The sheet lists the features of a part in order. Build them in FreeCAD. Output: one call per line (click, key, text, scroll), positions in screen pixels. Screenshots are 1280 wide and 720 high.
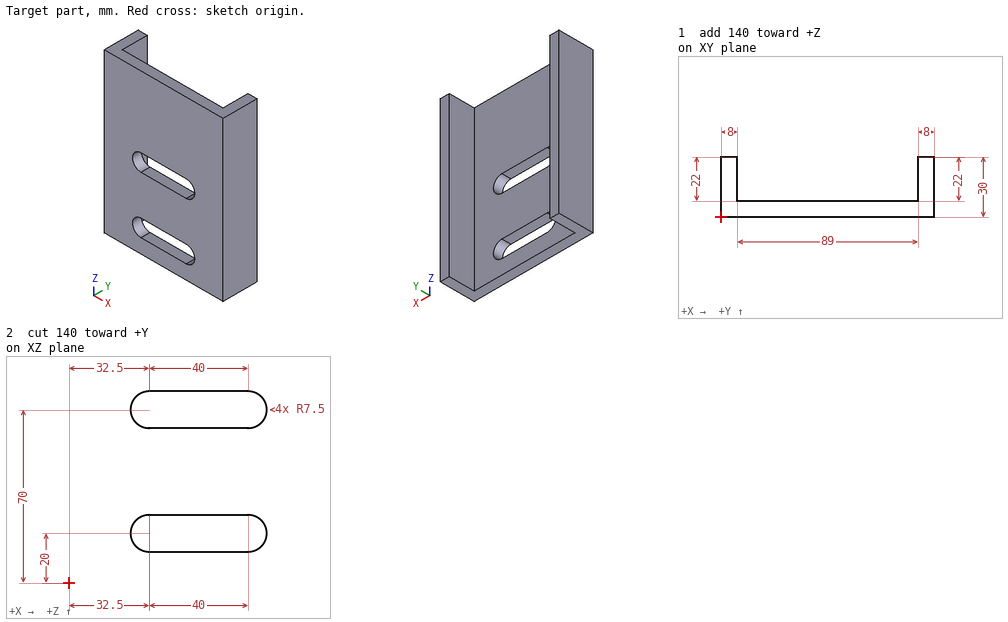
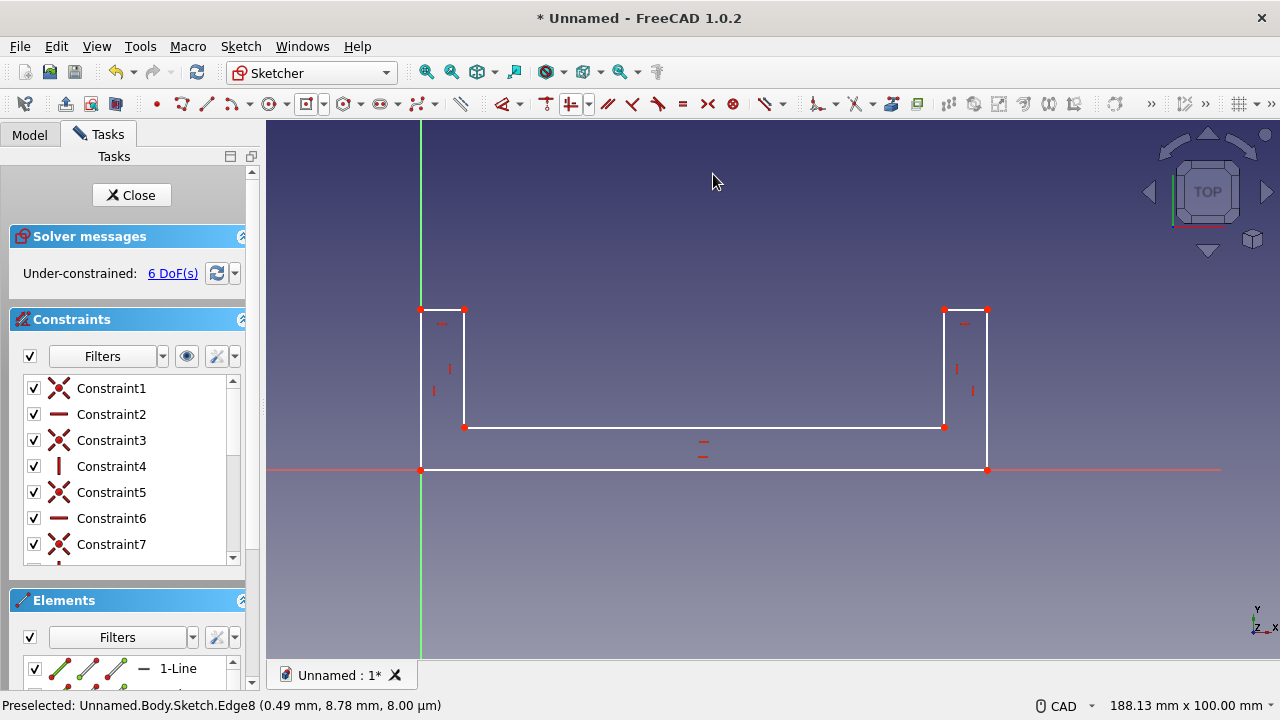
click(502, 104)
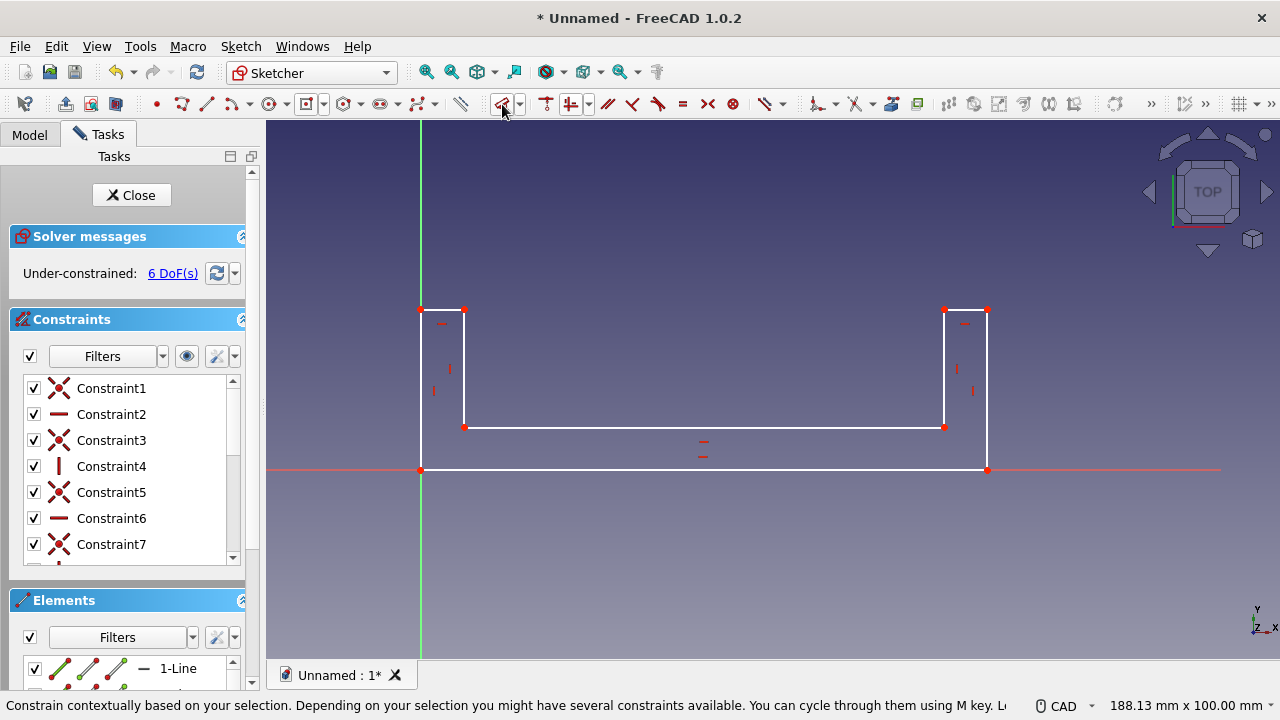
click(974, 310)
click(966, 276)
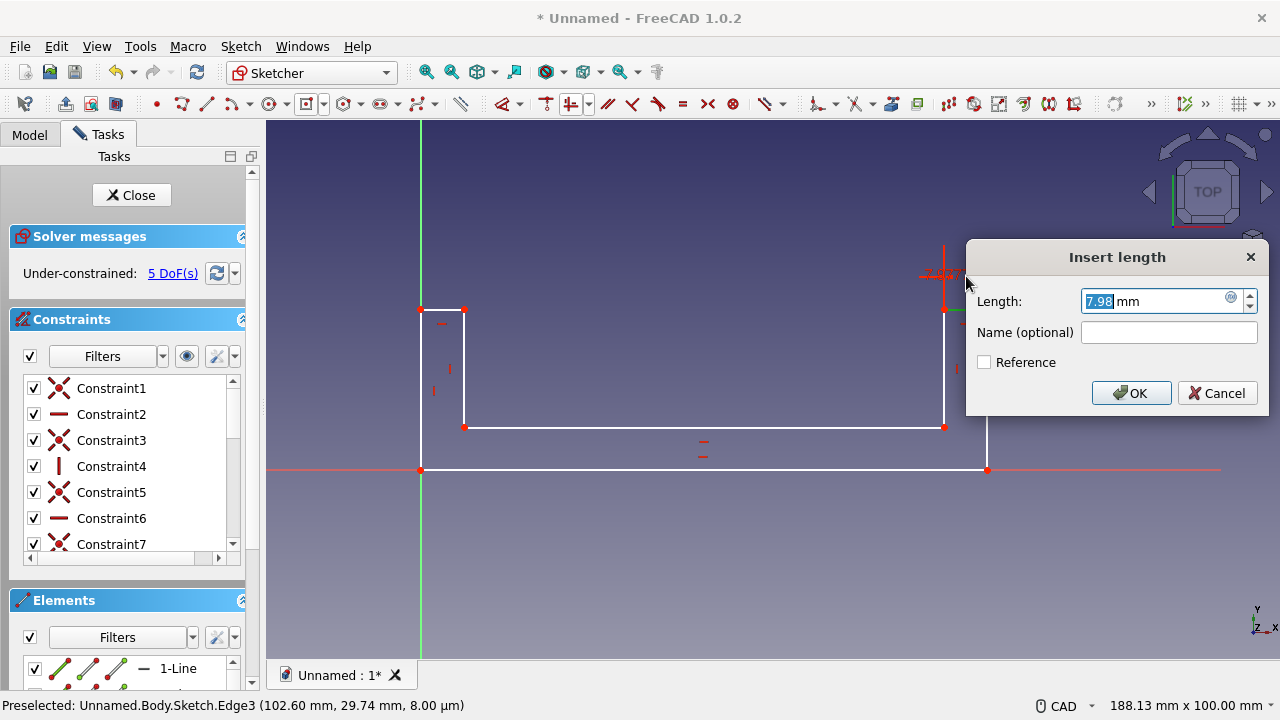
text(8)
key(Return)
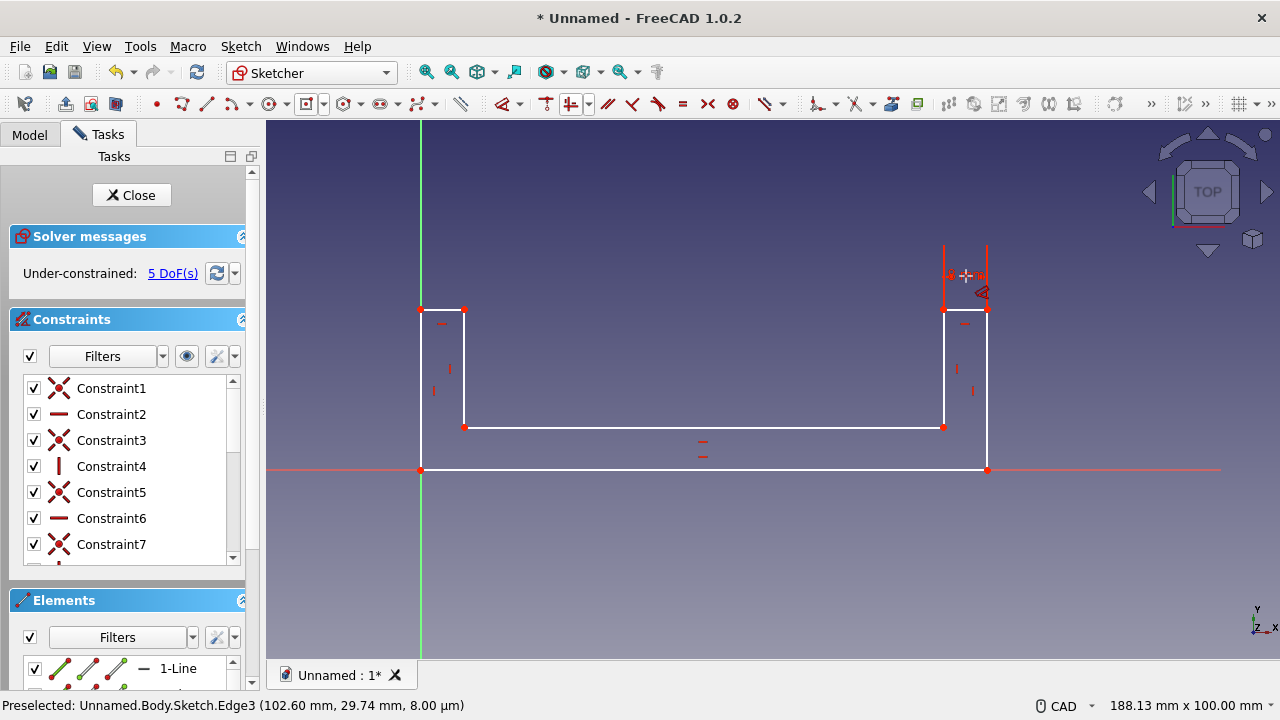
click(451, 310)
click(442, 276)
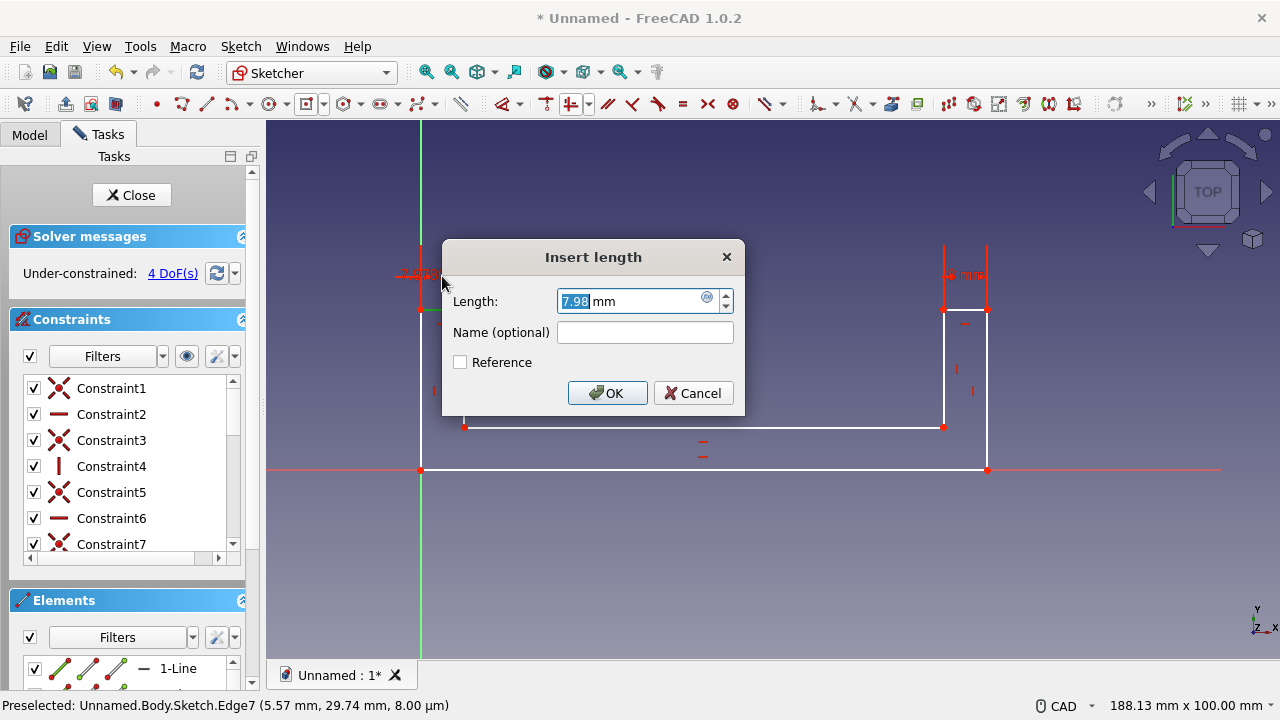
text(8)
key(Return)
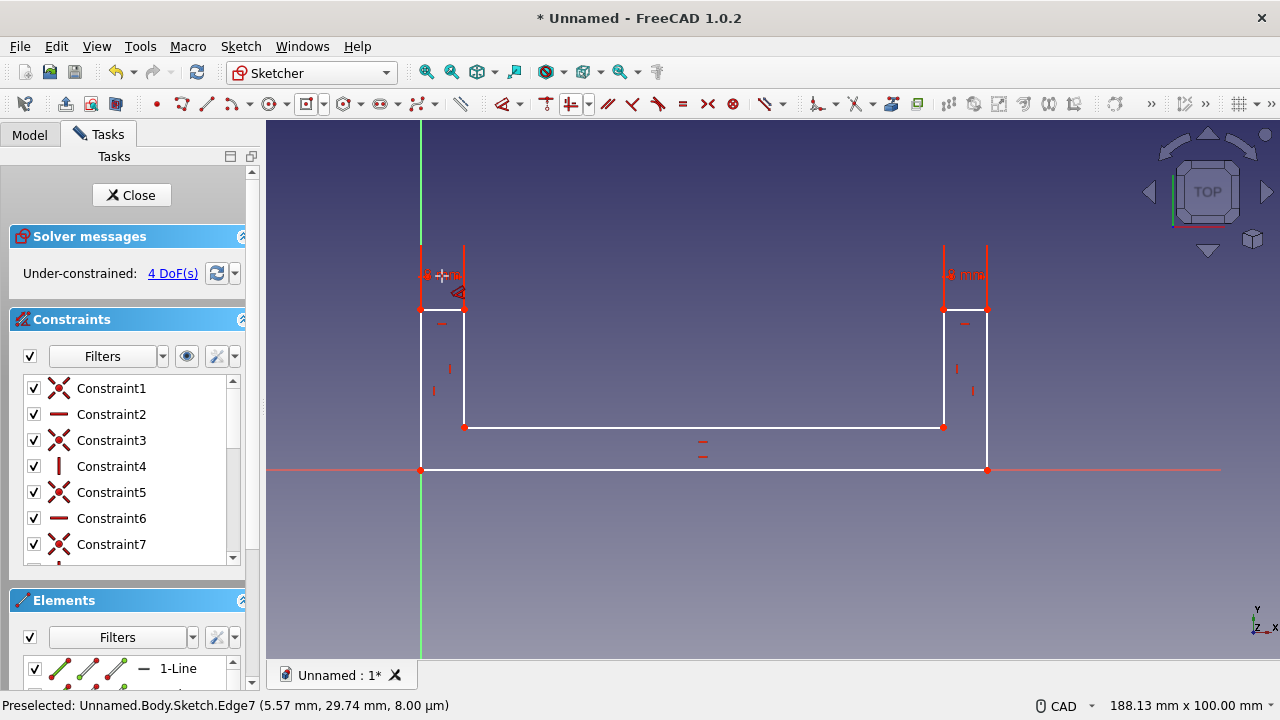
click(987, 422)
click(1021, 390)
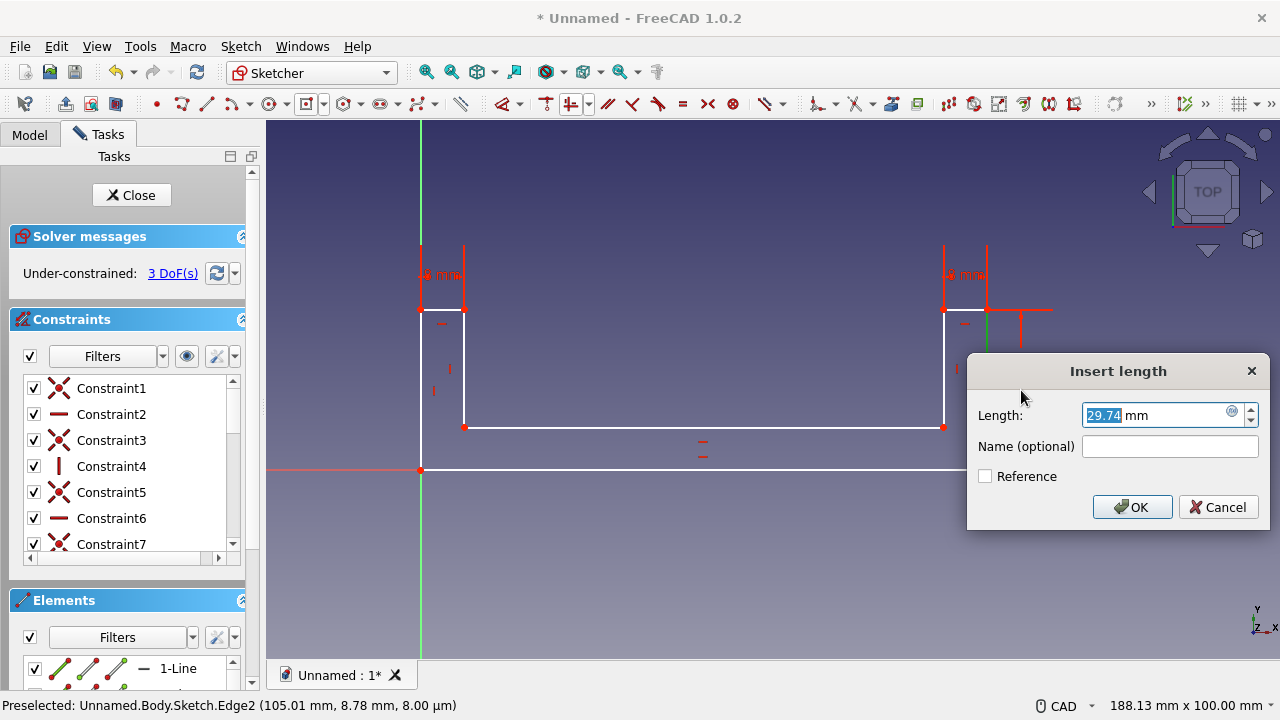
text(30)
key(Return)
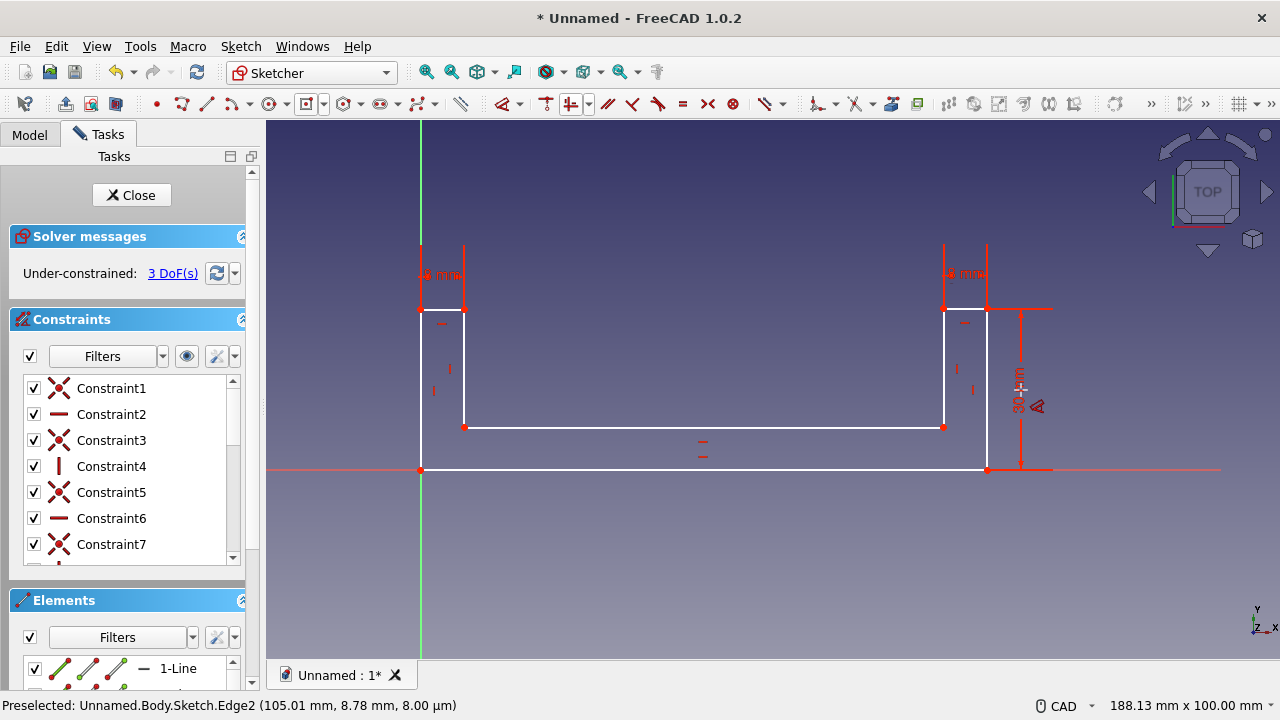
click(944, 344)
click(910, 368)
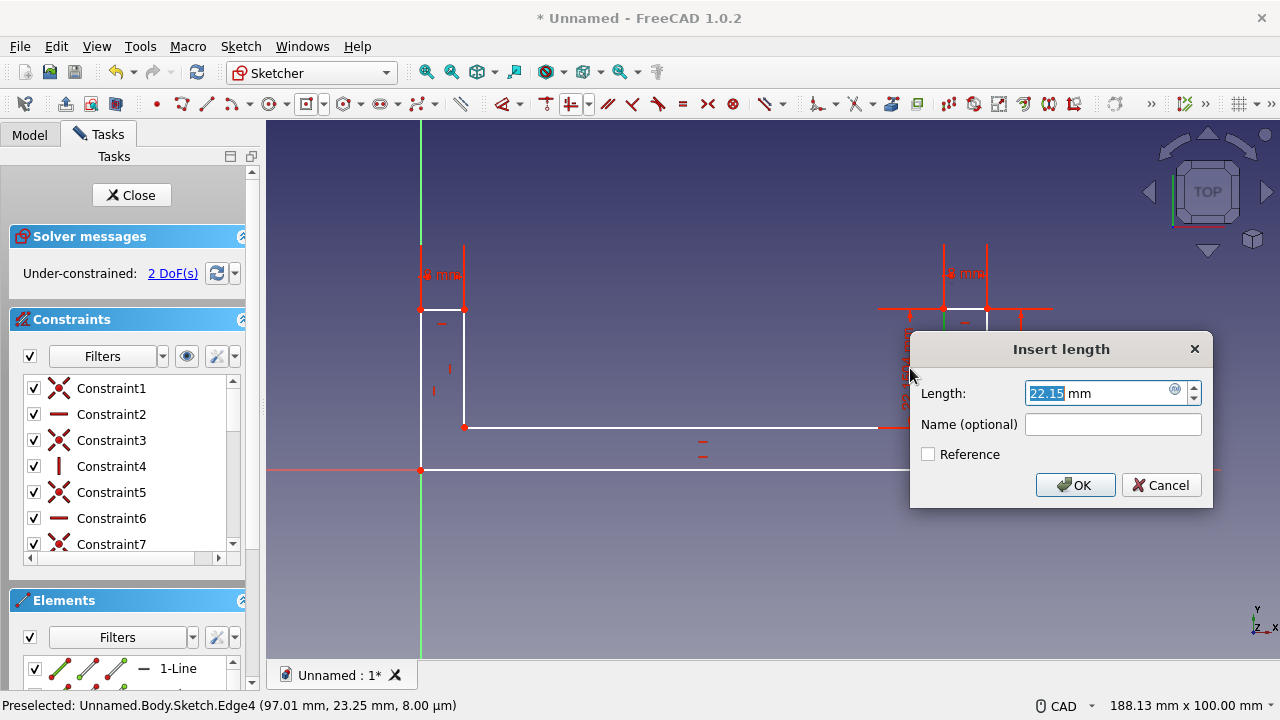
text(22)
key(Return)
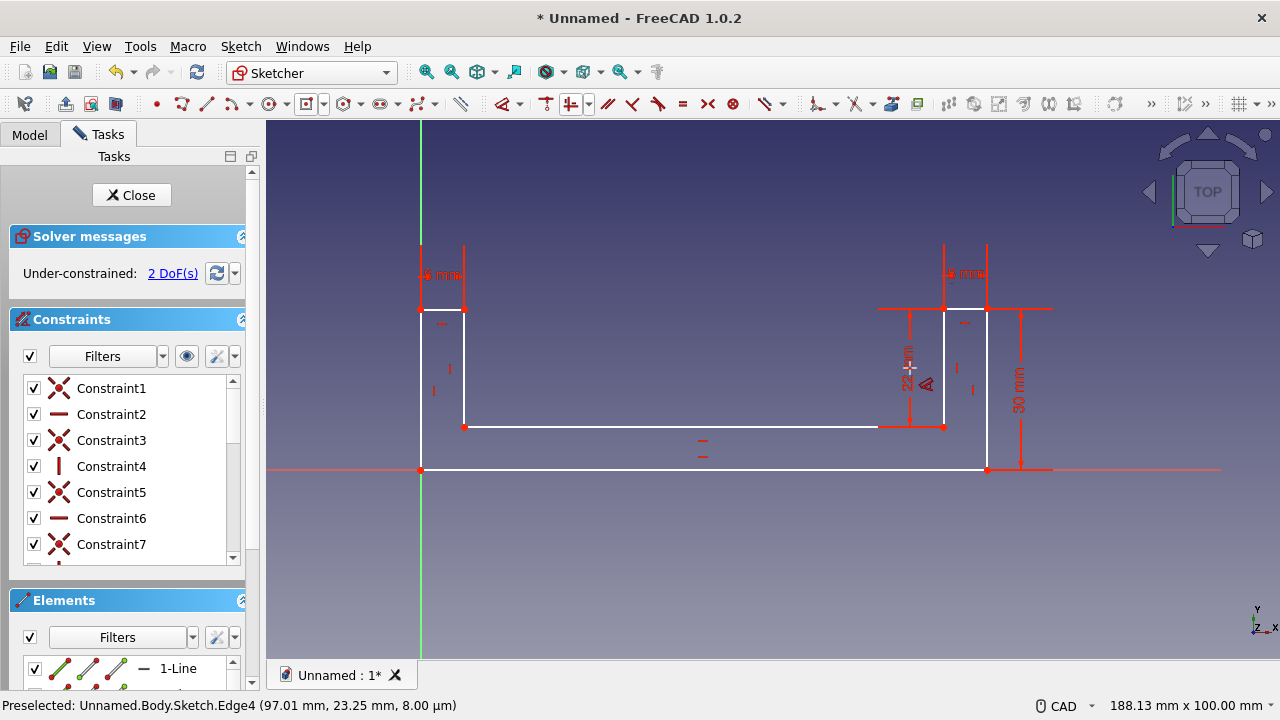
click(800, 427)
click(704, 393)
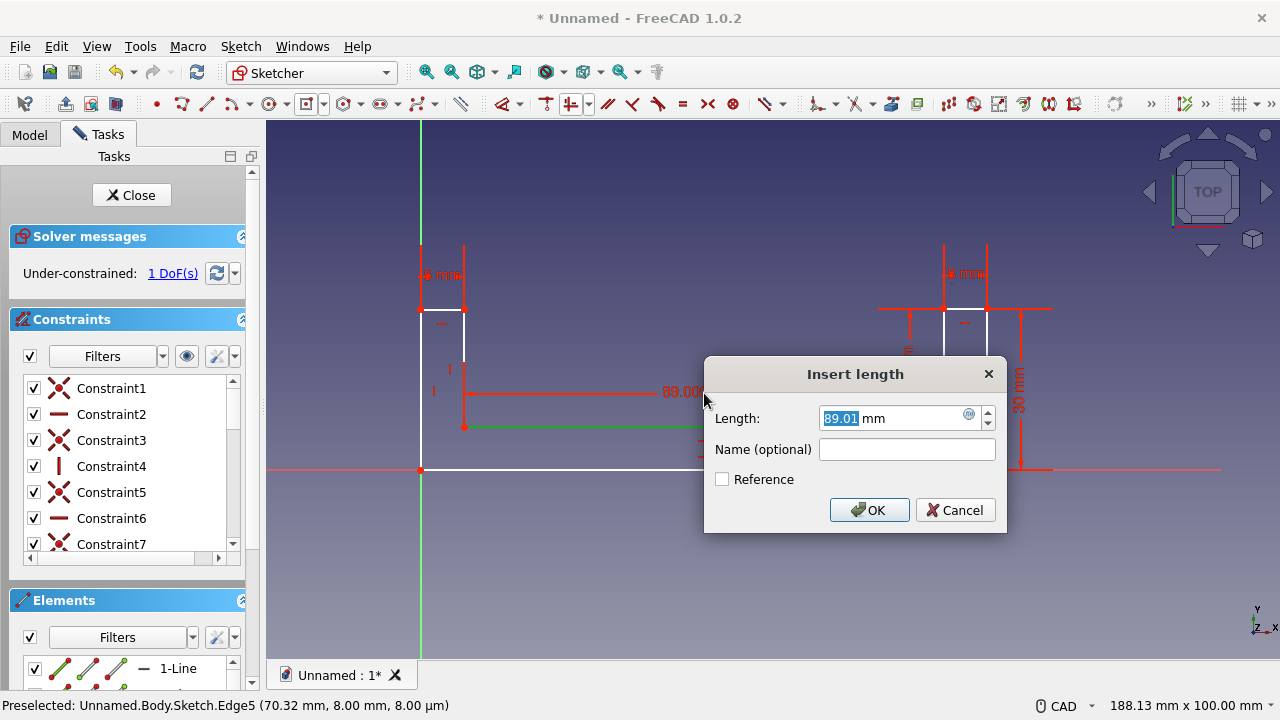
text(89)
key(Return)